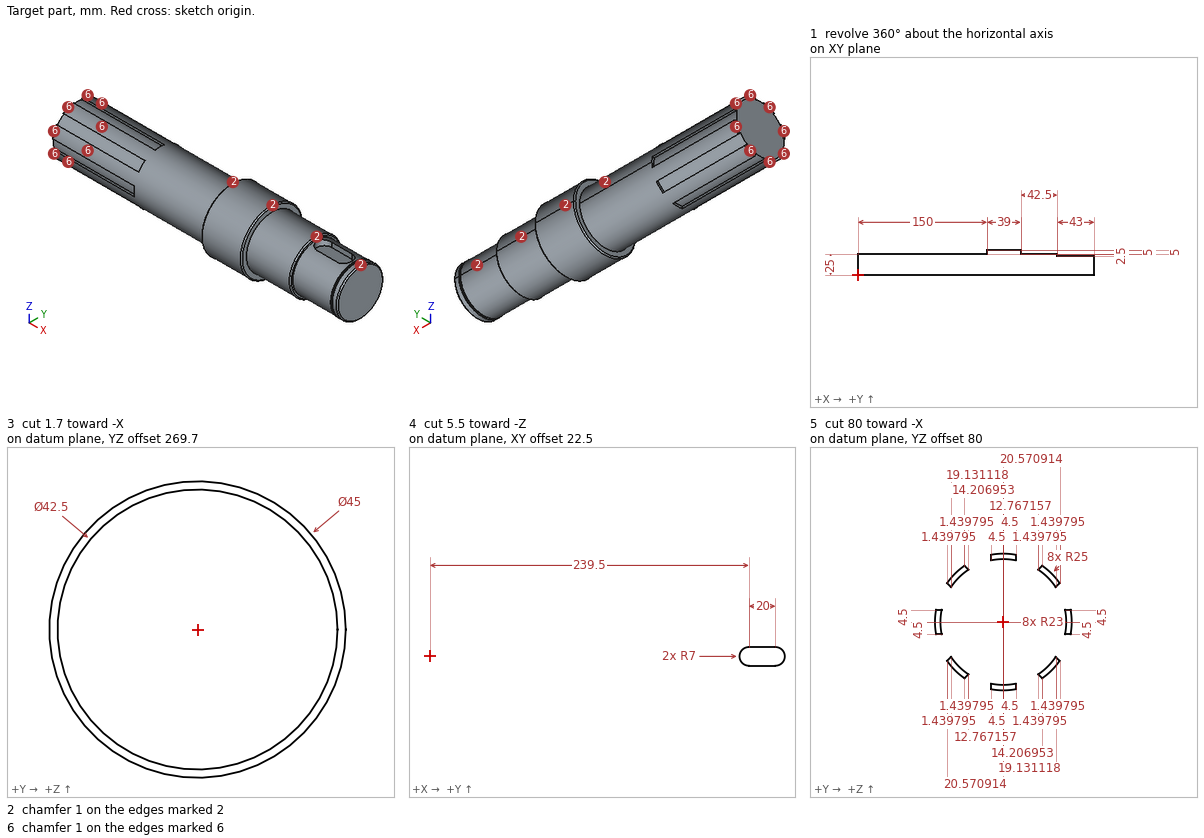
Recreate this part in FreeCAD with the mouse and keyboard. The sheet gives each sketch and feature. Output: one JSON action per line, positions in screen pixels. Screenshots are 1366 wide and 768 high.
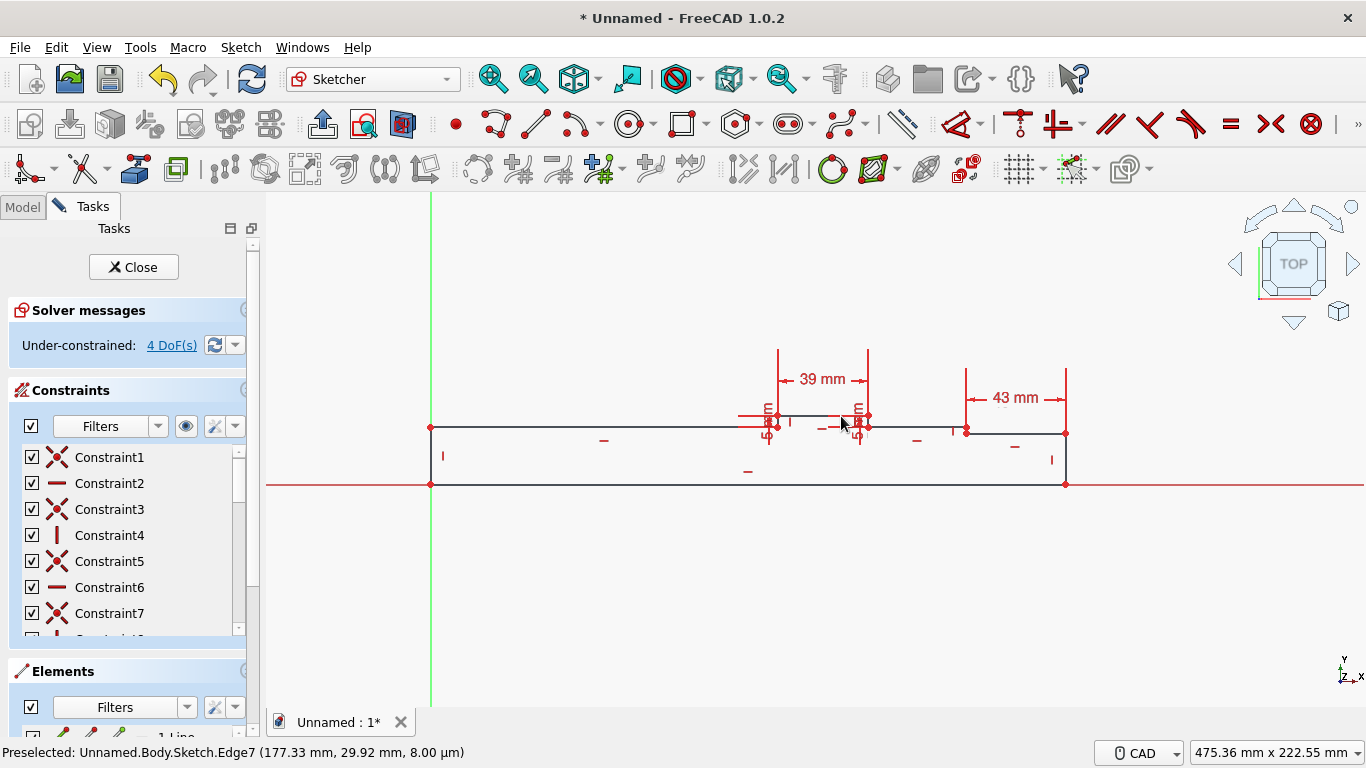
{"action": "left_click", "coordinate": [431, 444]}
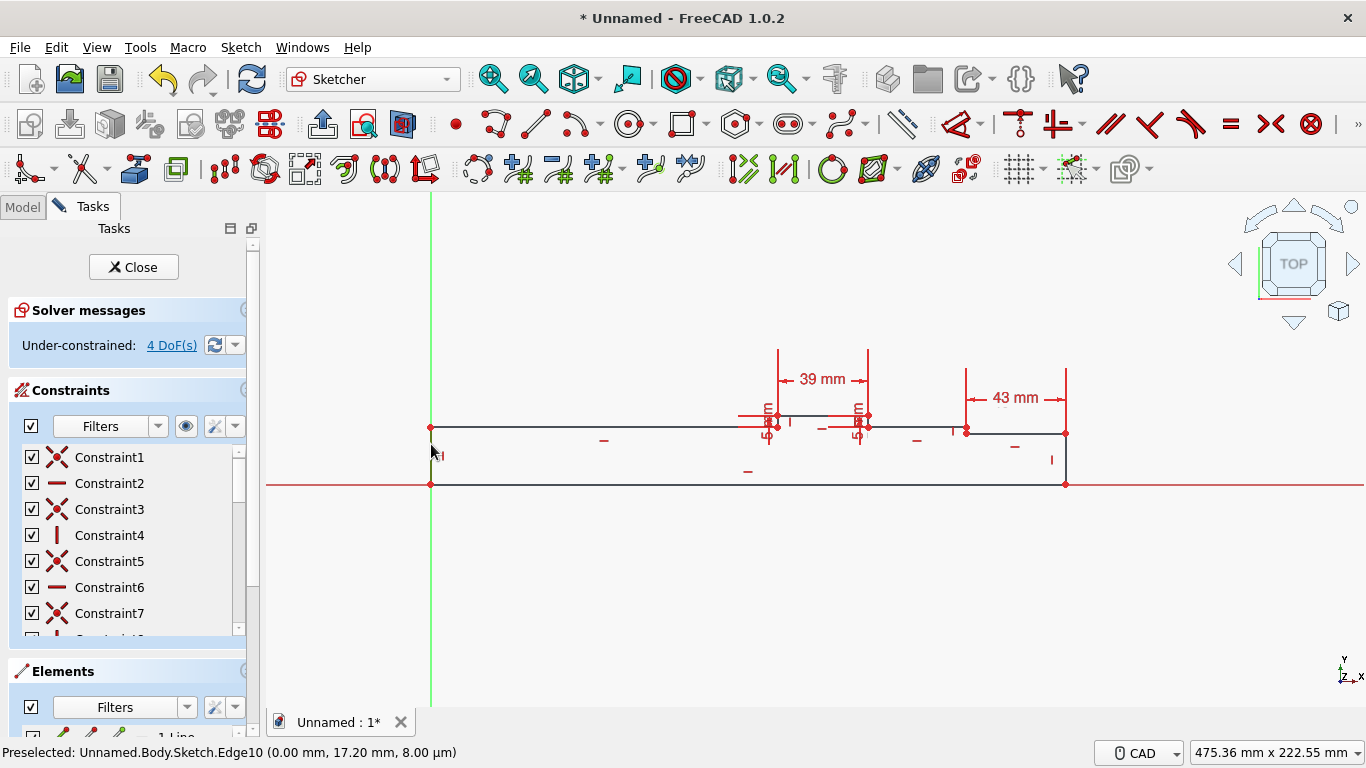
{"action": "left_click", "coordinate": [982, 124]}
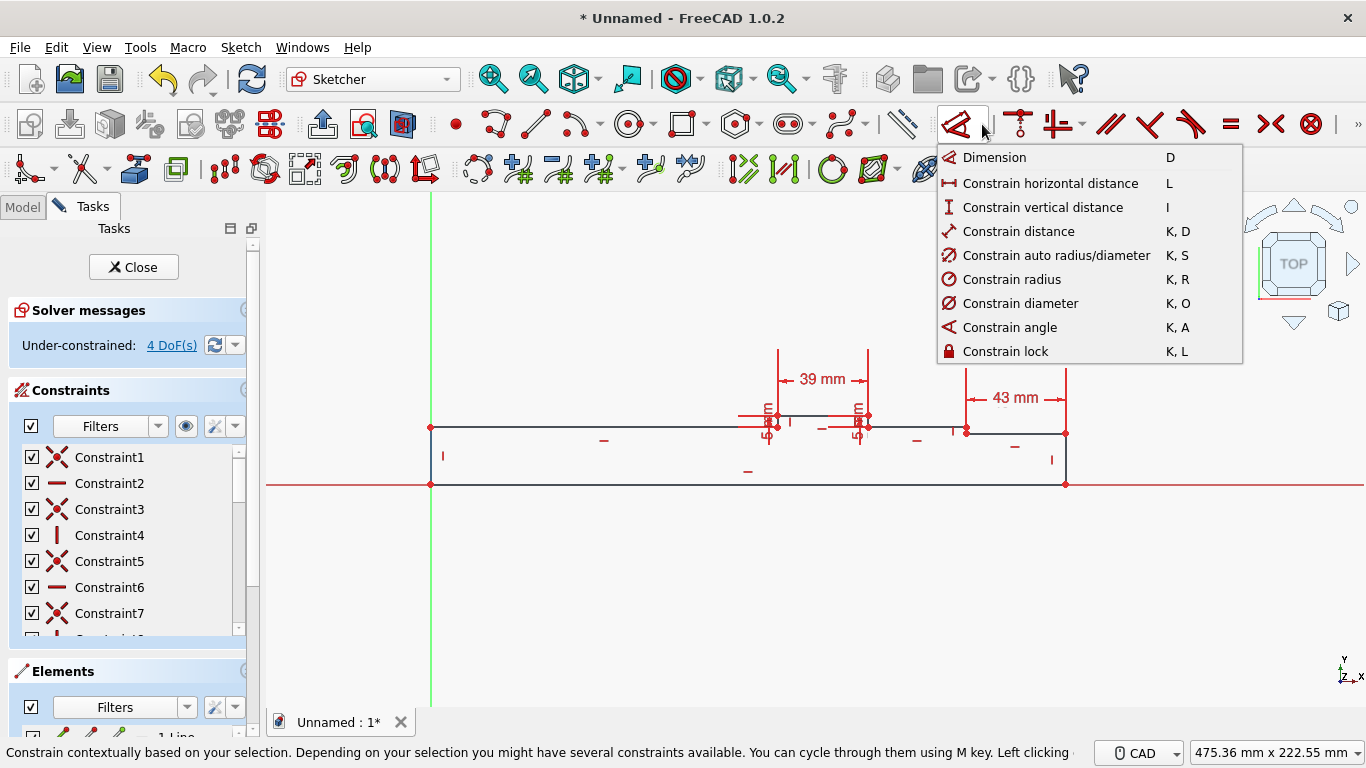
{"action": "left_click", "coordinate": [1090, 207]}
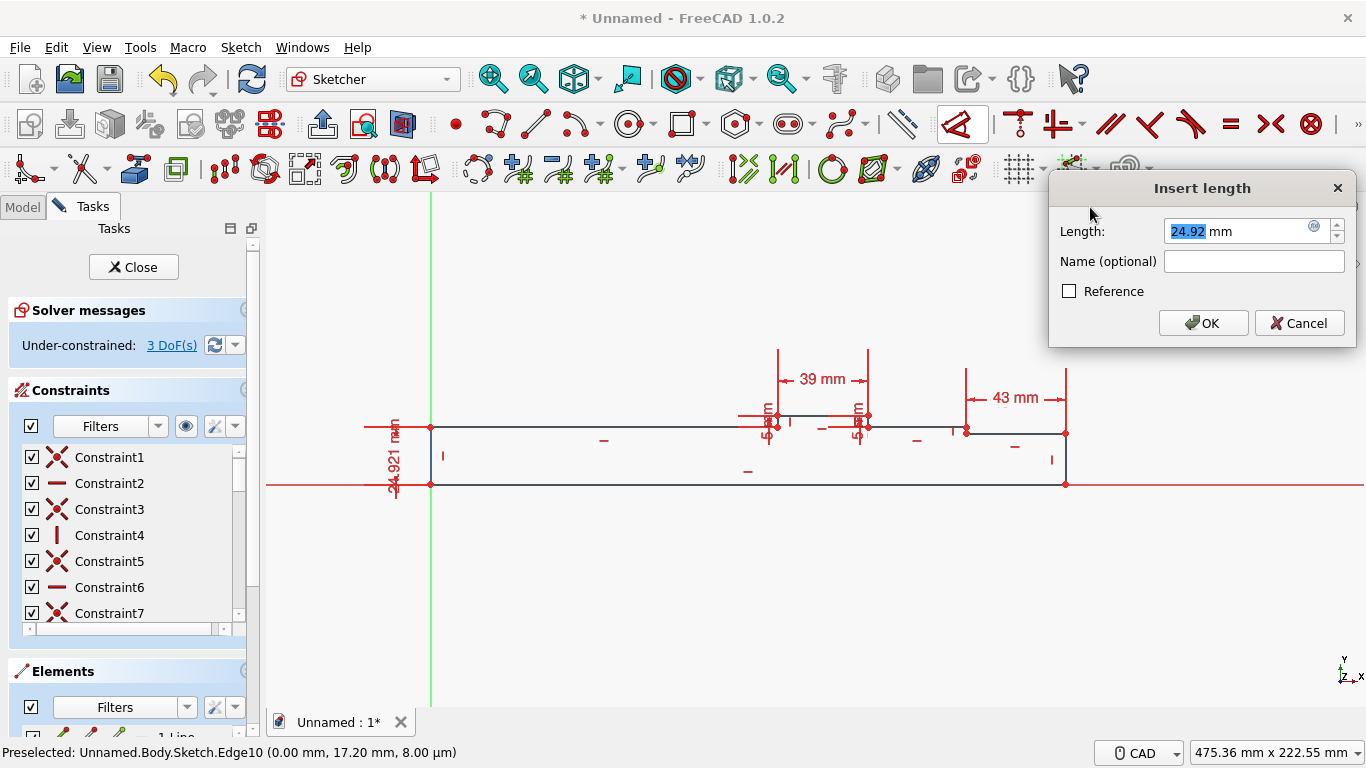
{"action": "type", "text": "25"}
{"action": "key", "text": "Return"}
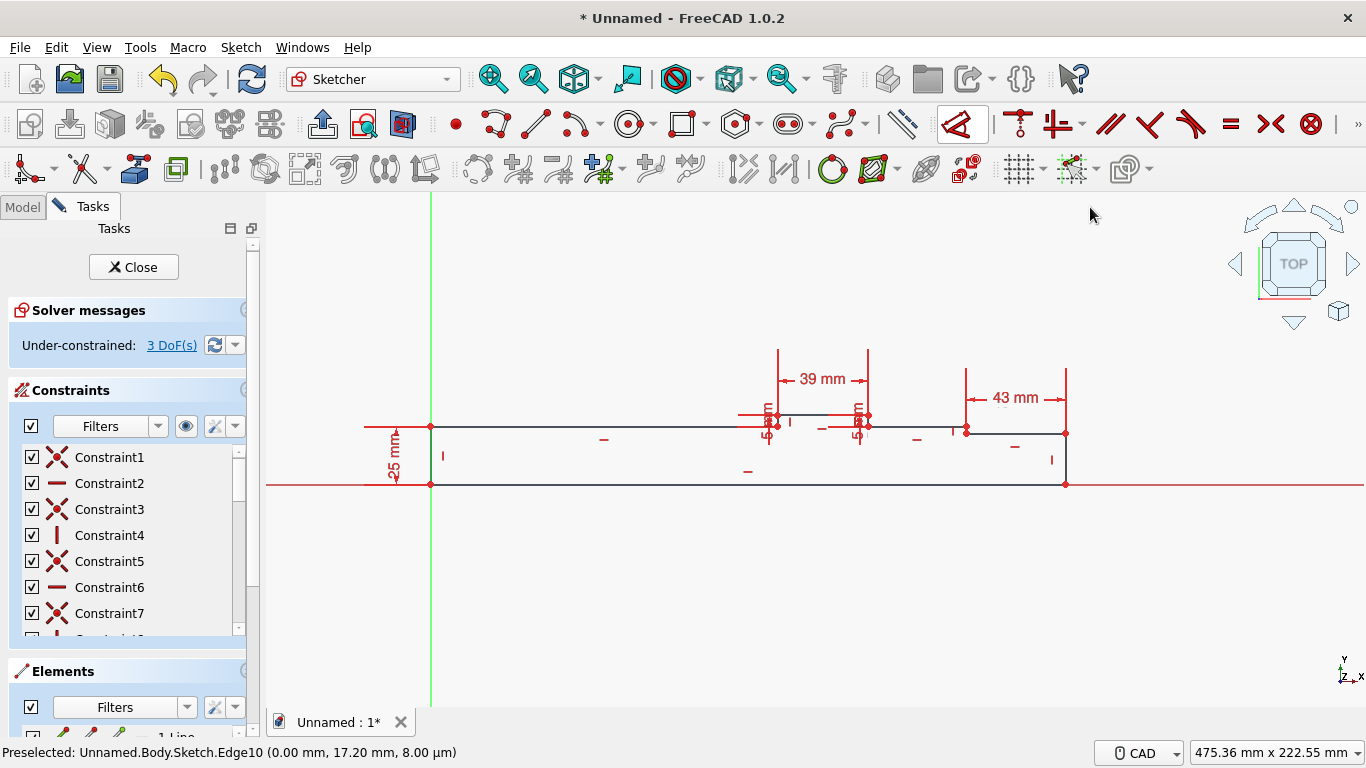
{"action": "scroll", "coordinate": [966, 430], "scroll_direction": "up", "scroll_amount": 10}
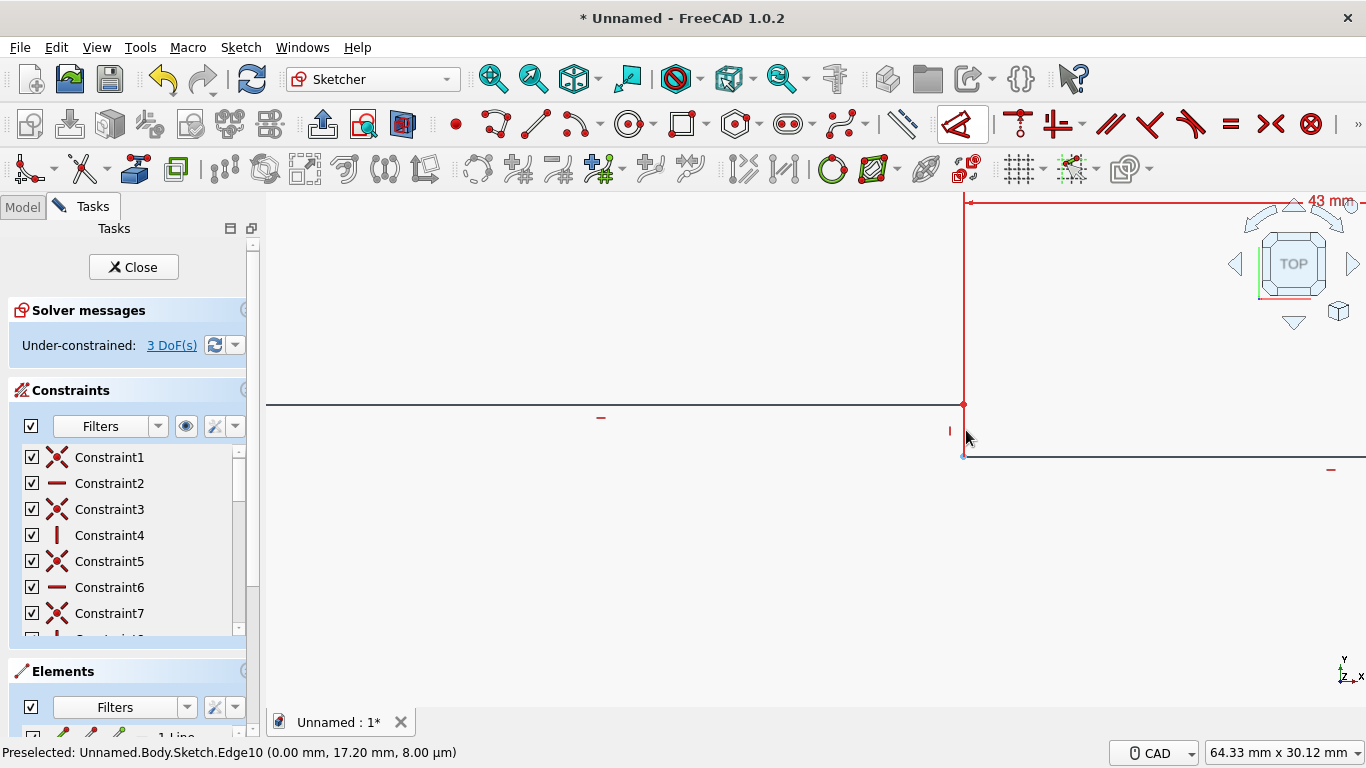
{"action": "left_click", "coordinate": [964, 431]}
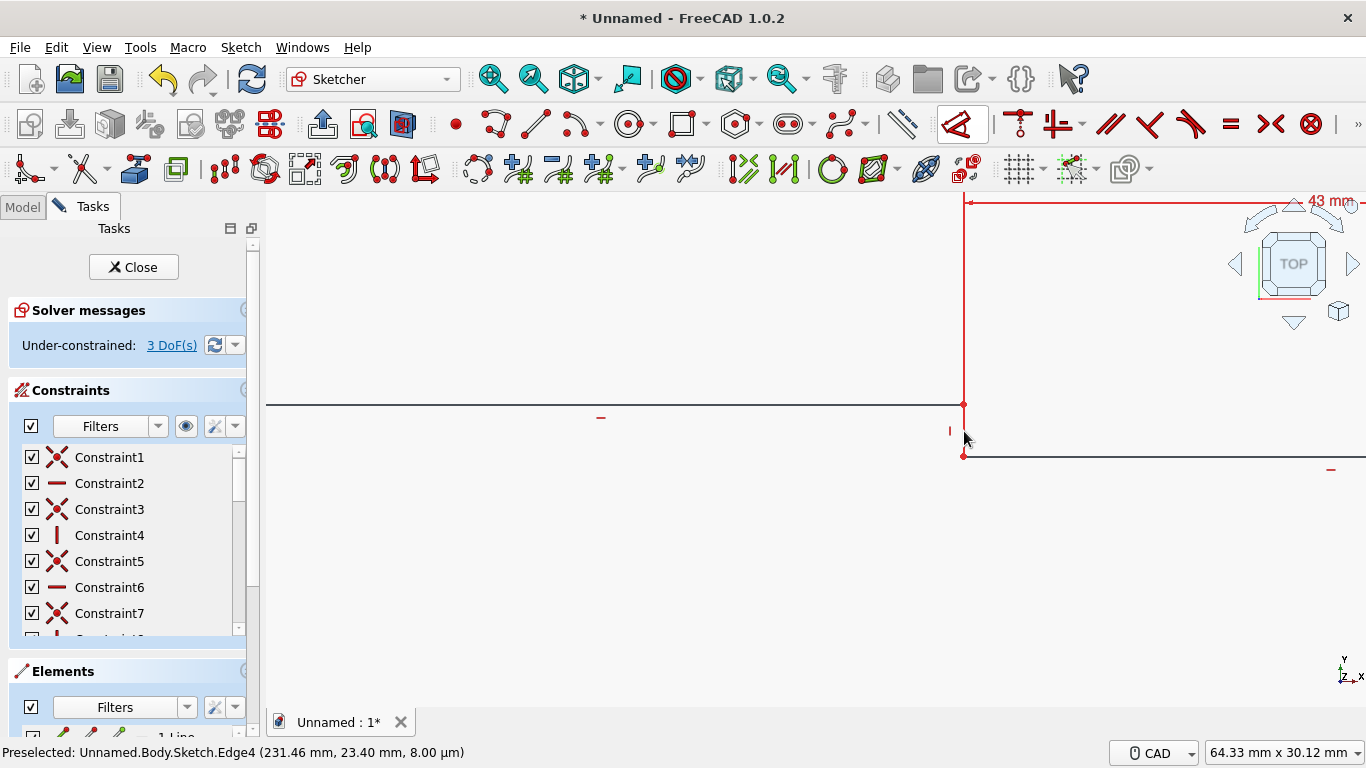
{"action": "left_click", "coordinate": [982, 124]}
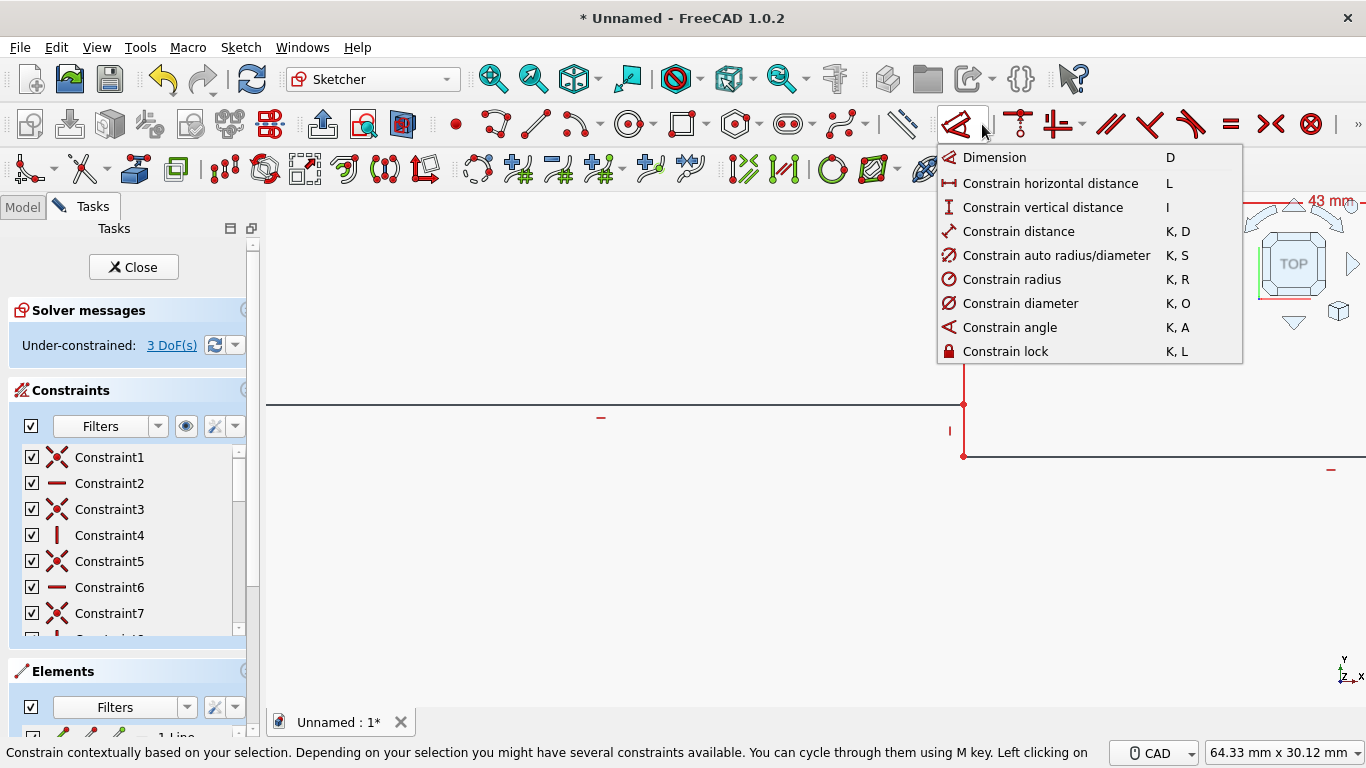
{"action": "left_click", "coordinate": [1090, 207]}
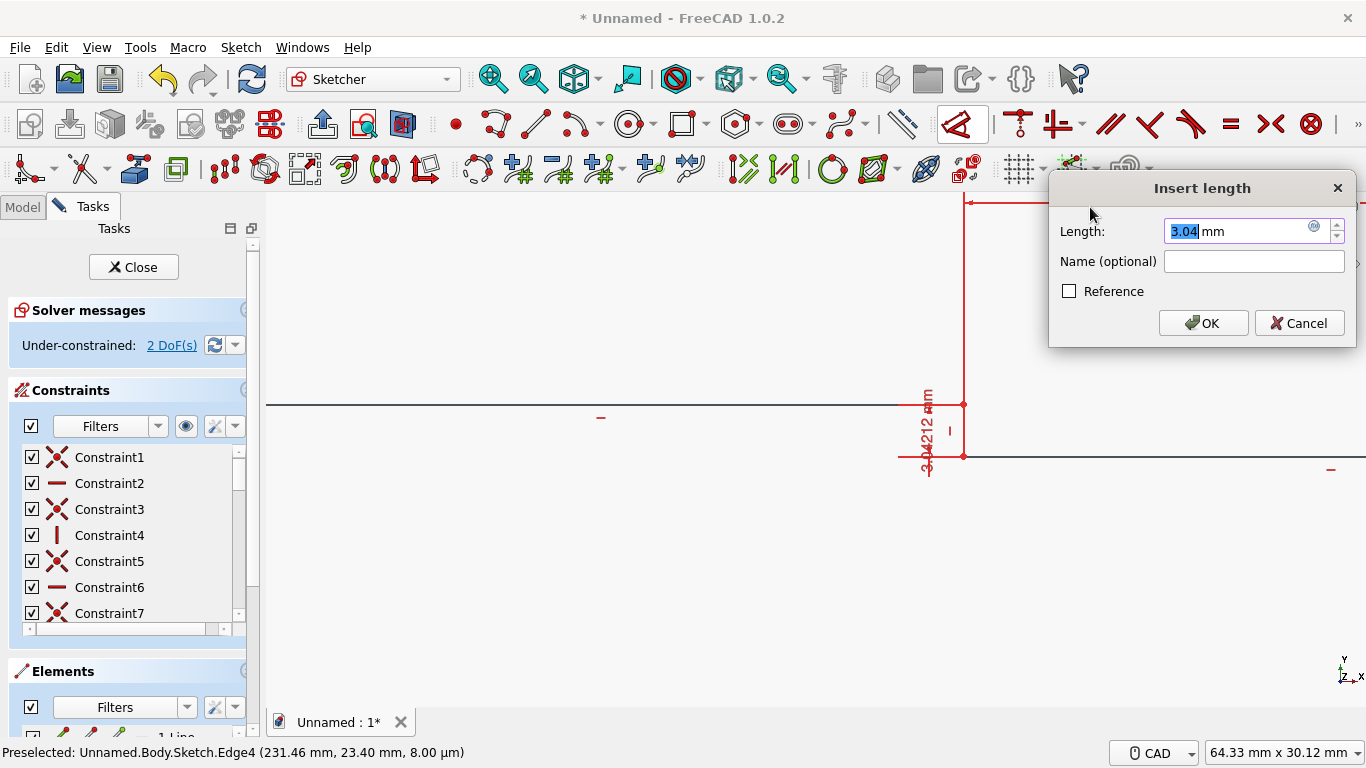
{"action": "type", "text": "2.5"}
{"action": "key", "text": "Return"}